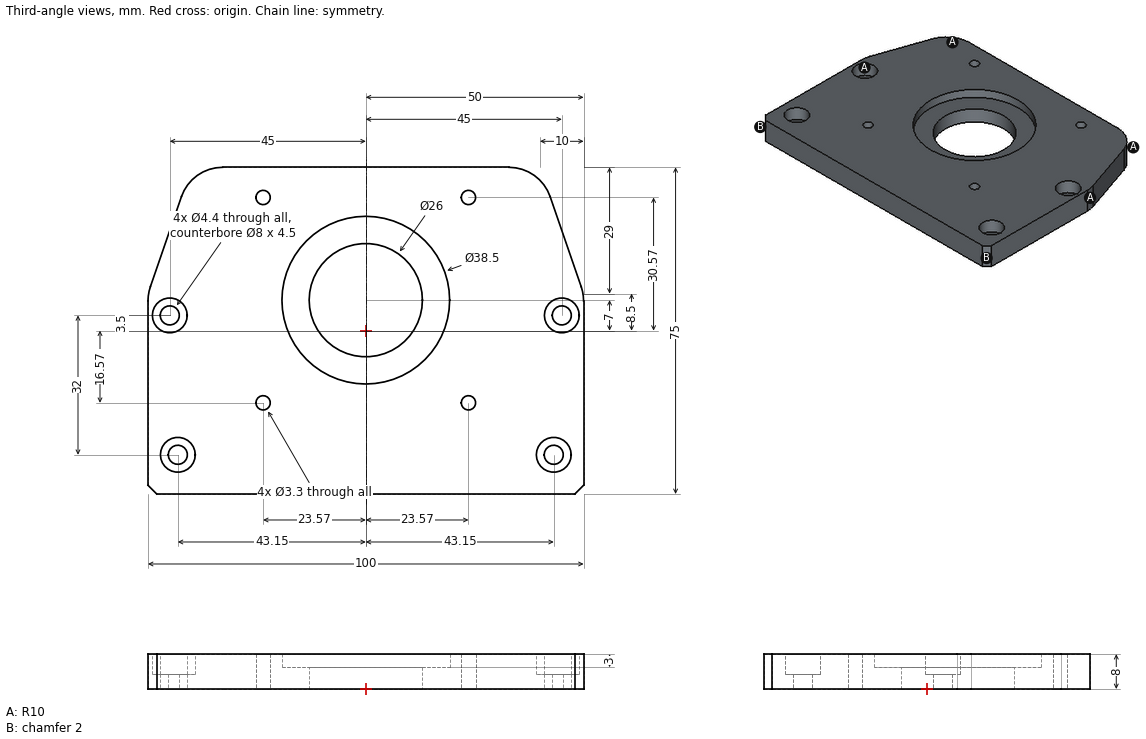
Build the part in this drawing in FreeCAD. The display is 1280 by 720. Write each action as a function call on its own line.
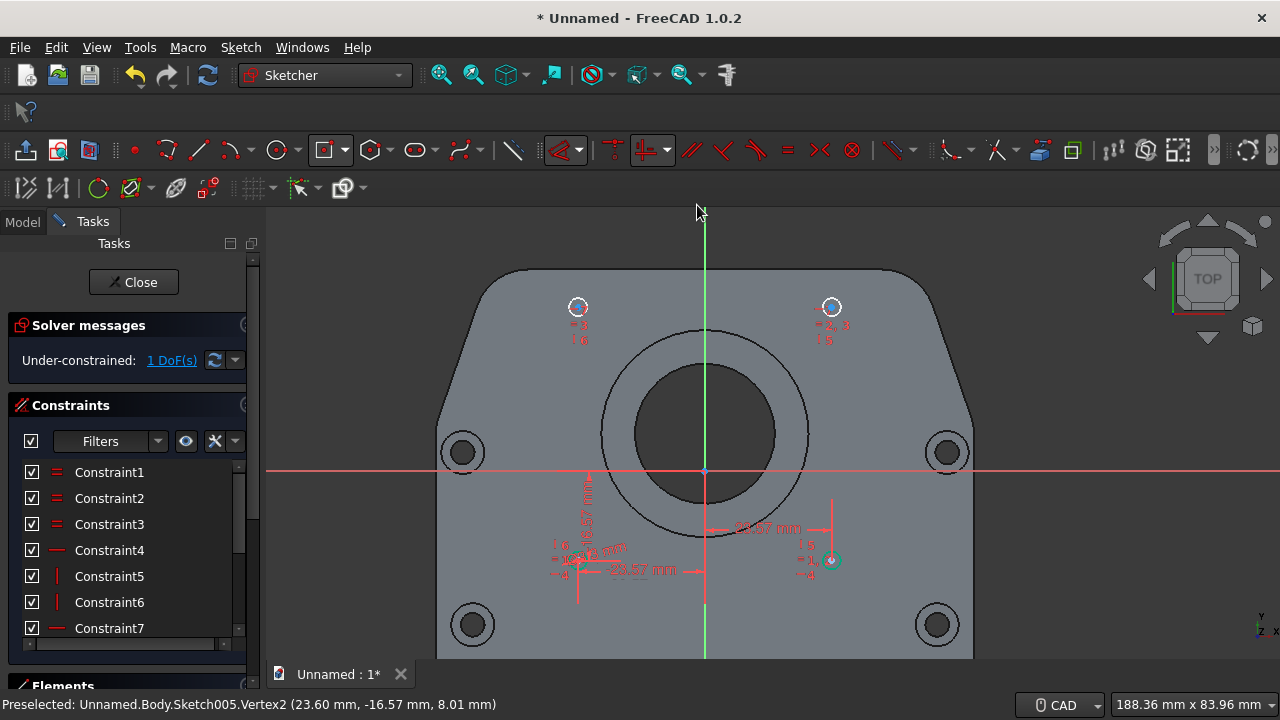
click(832, 307)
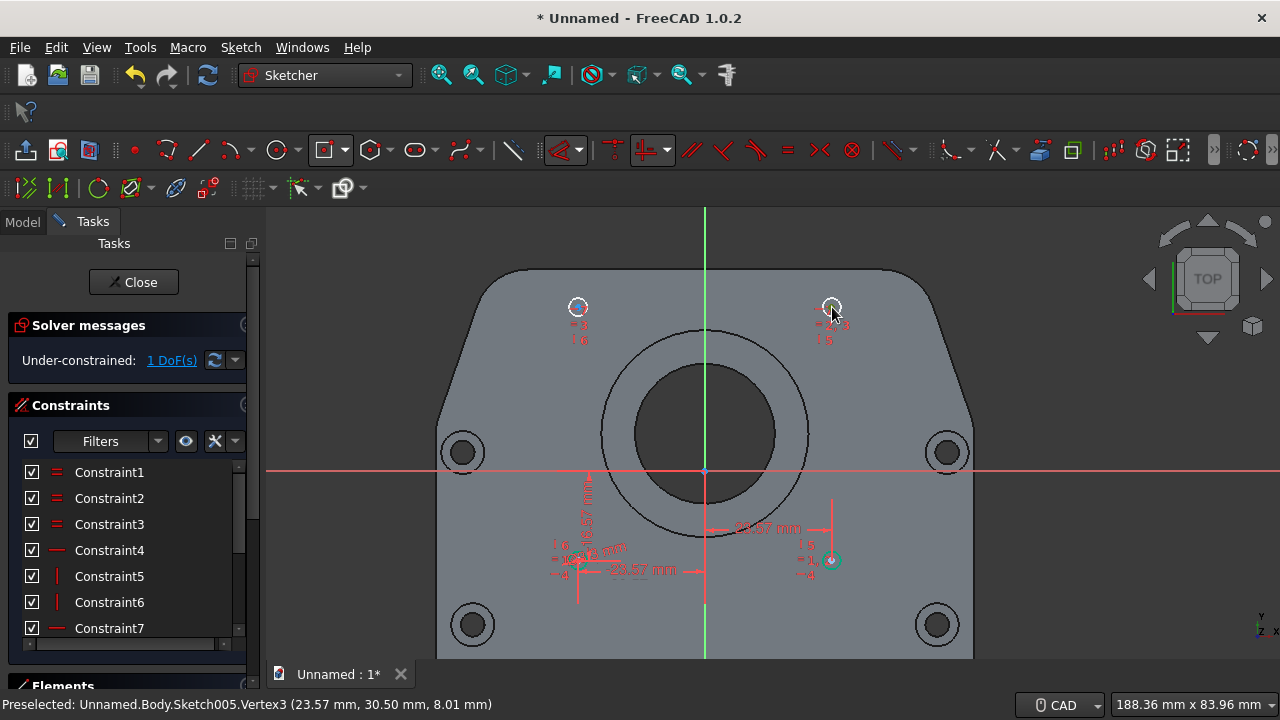
key(i)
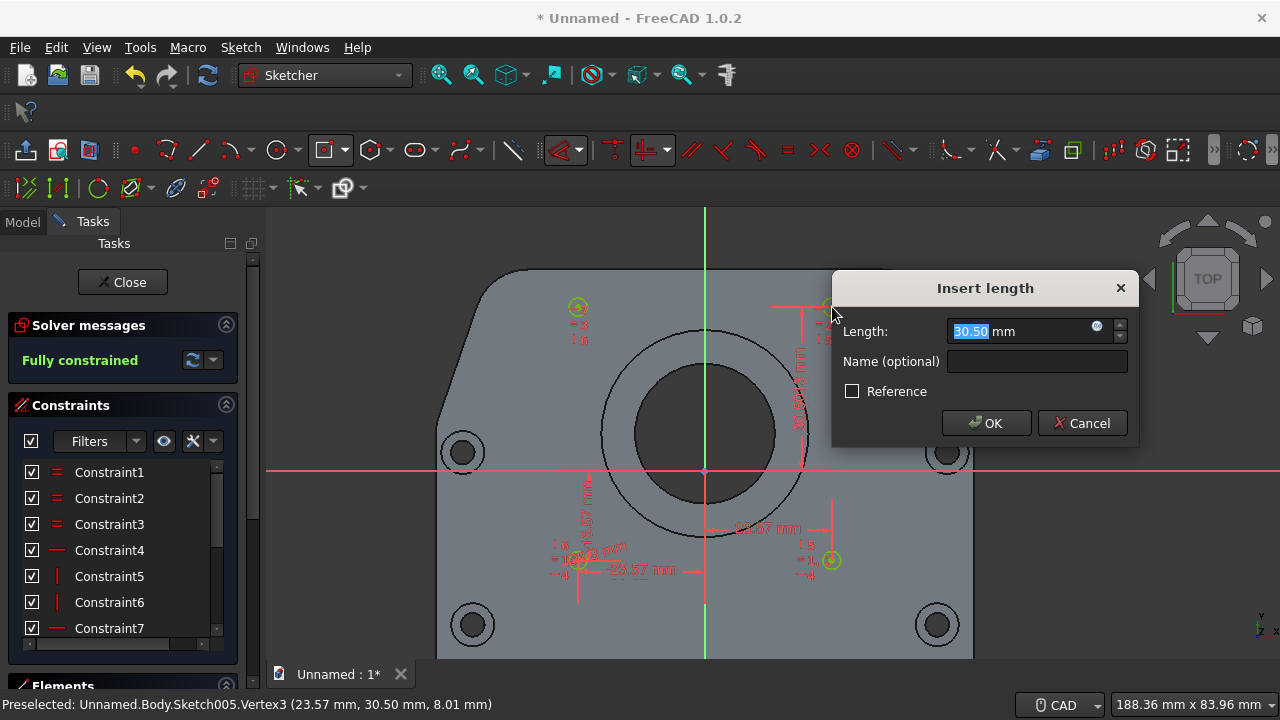
text(30.57)
key(Return)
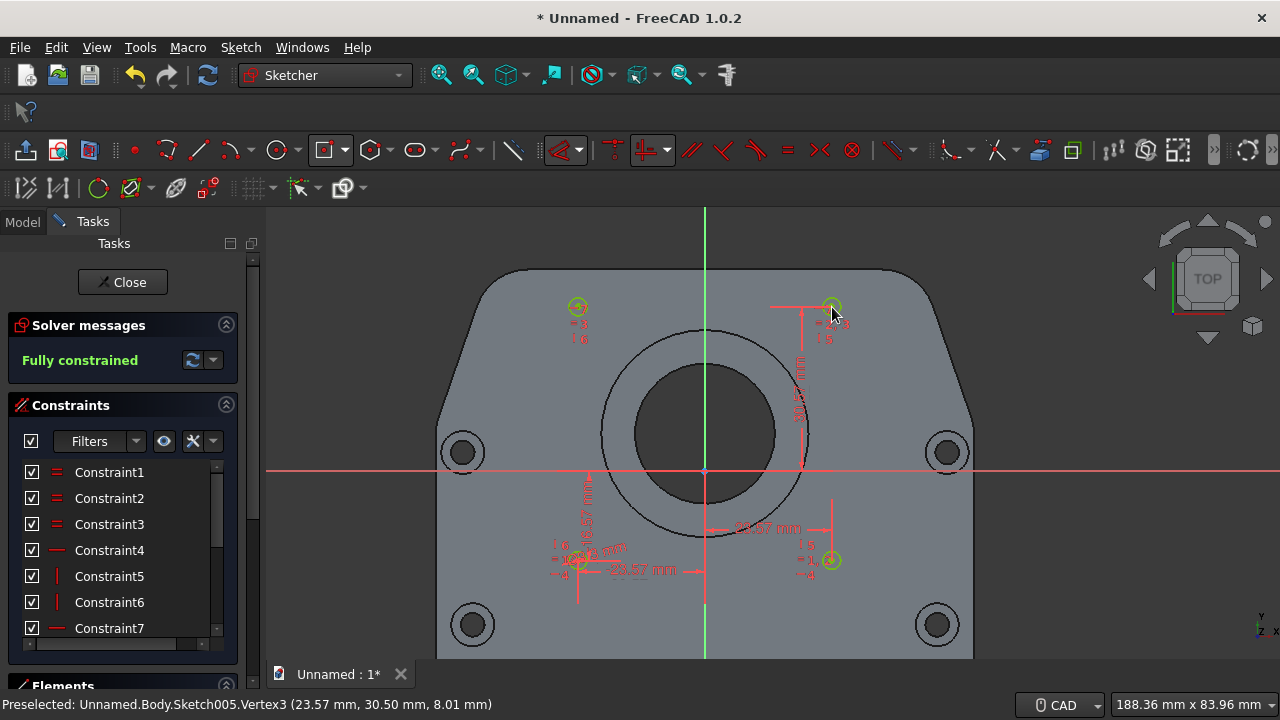
click(123, 282)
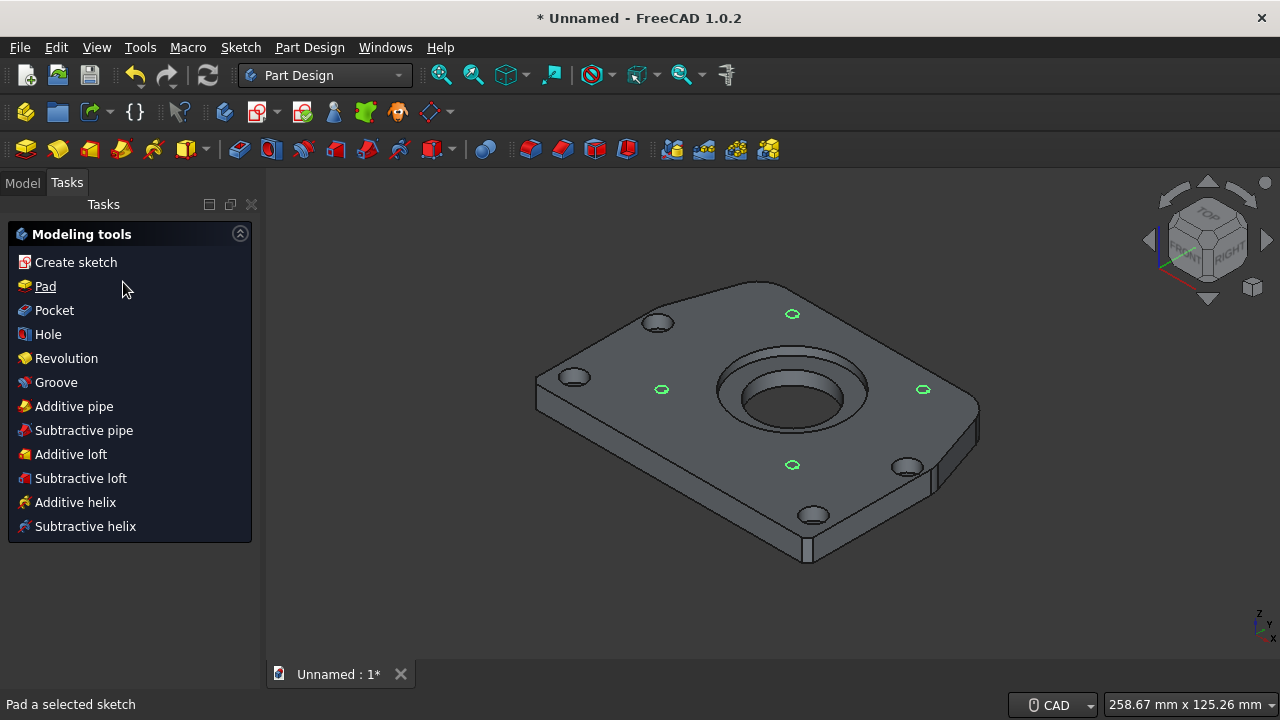
click(272, 150)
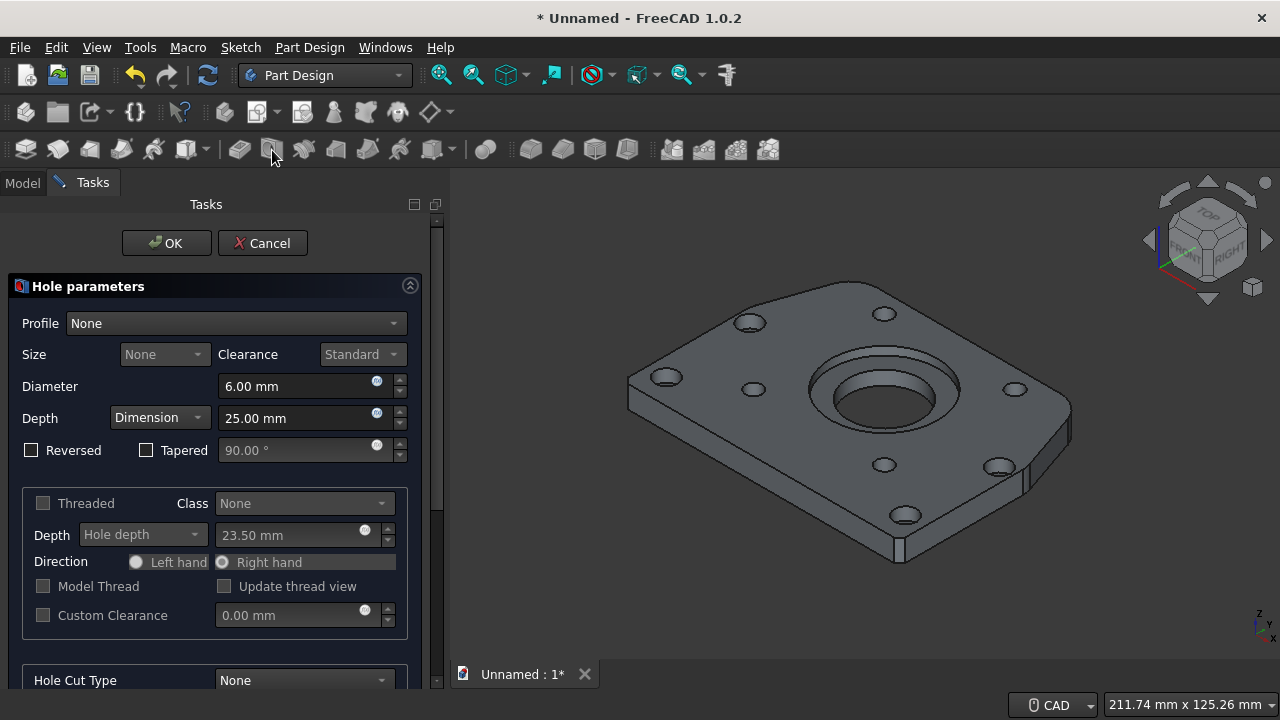
triple_click(305, 386)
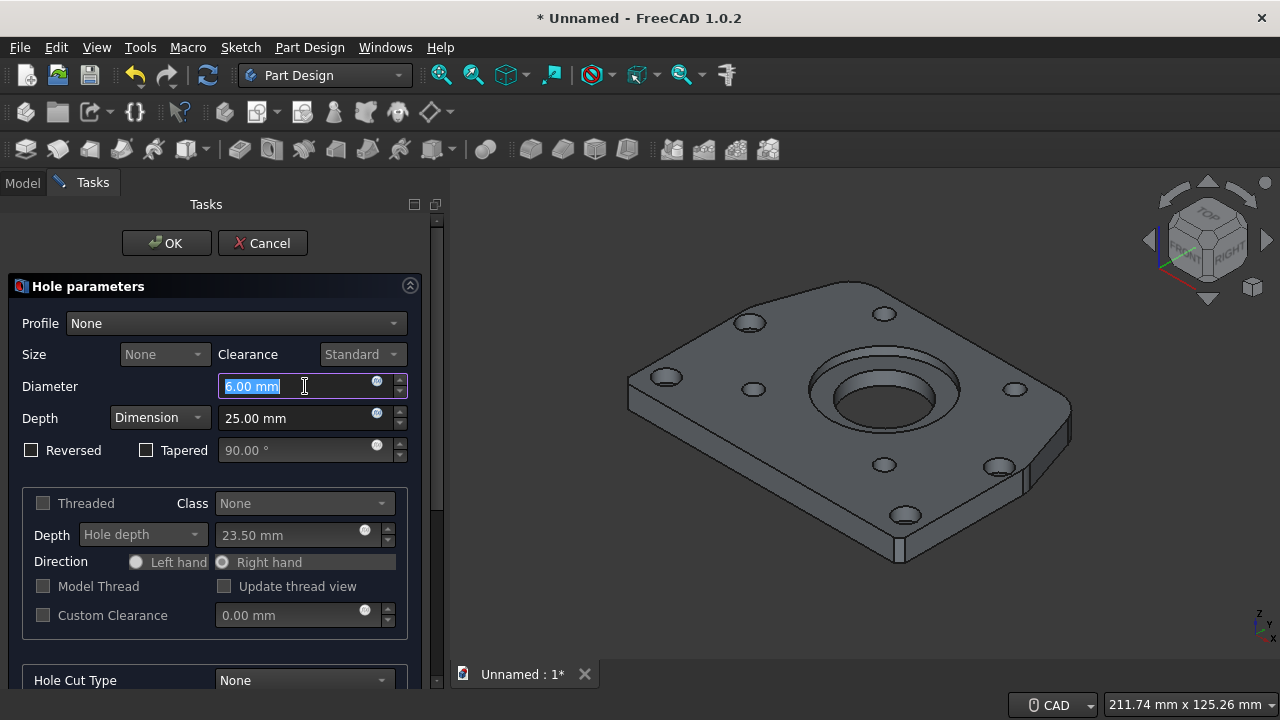
text(3.3)
key(Tab)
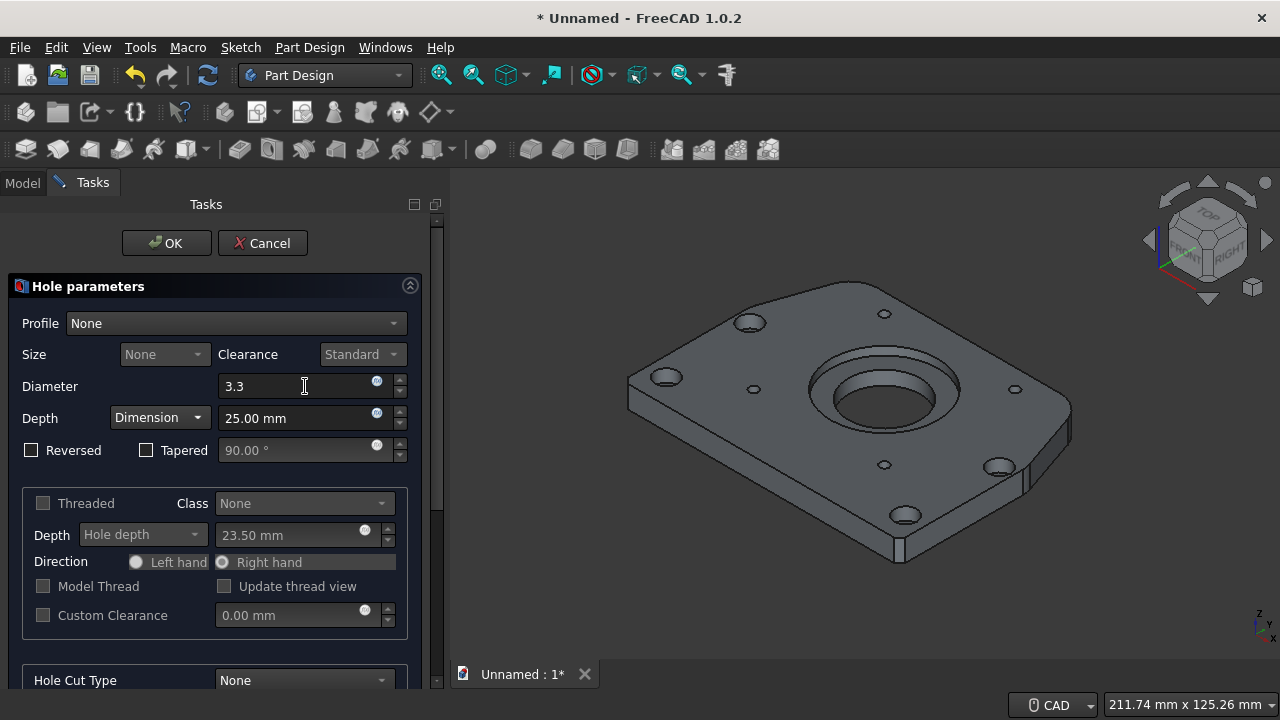
click(161, 418)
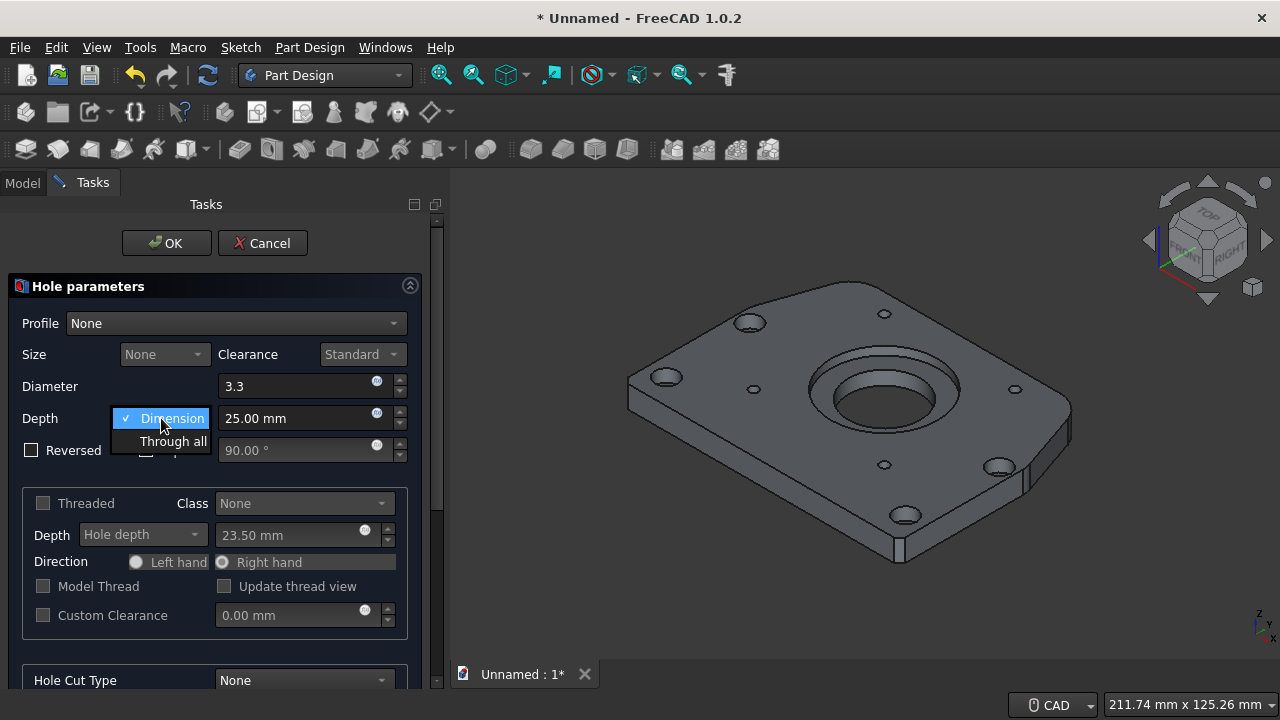
click(160, 442)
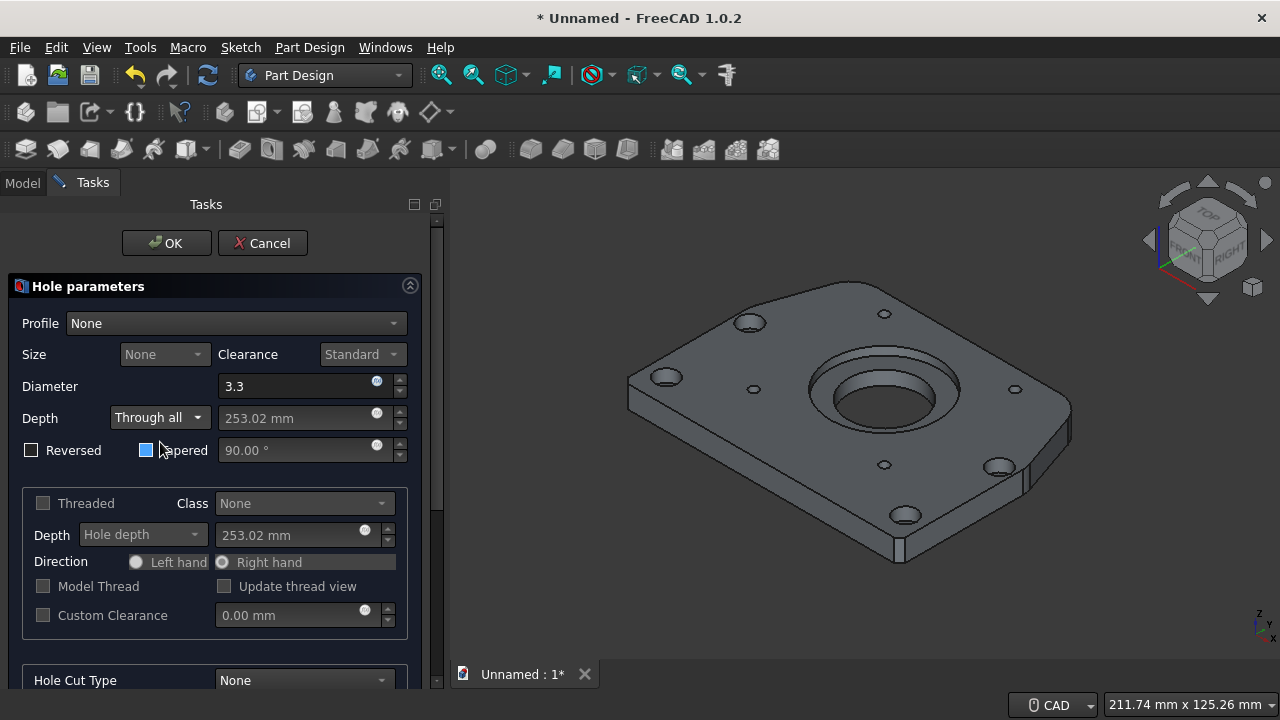
click(167, 243)